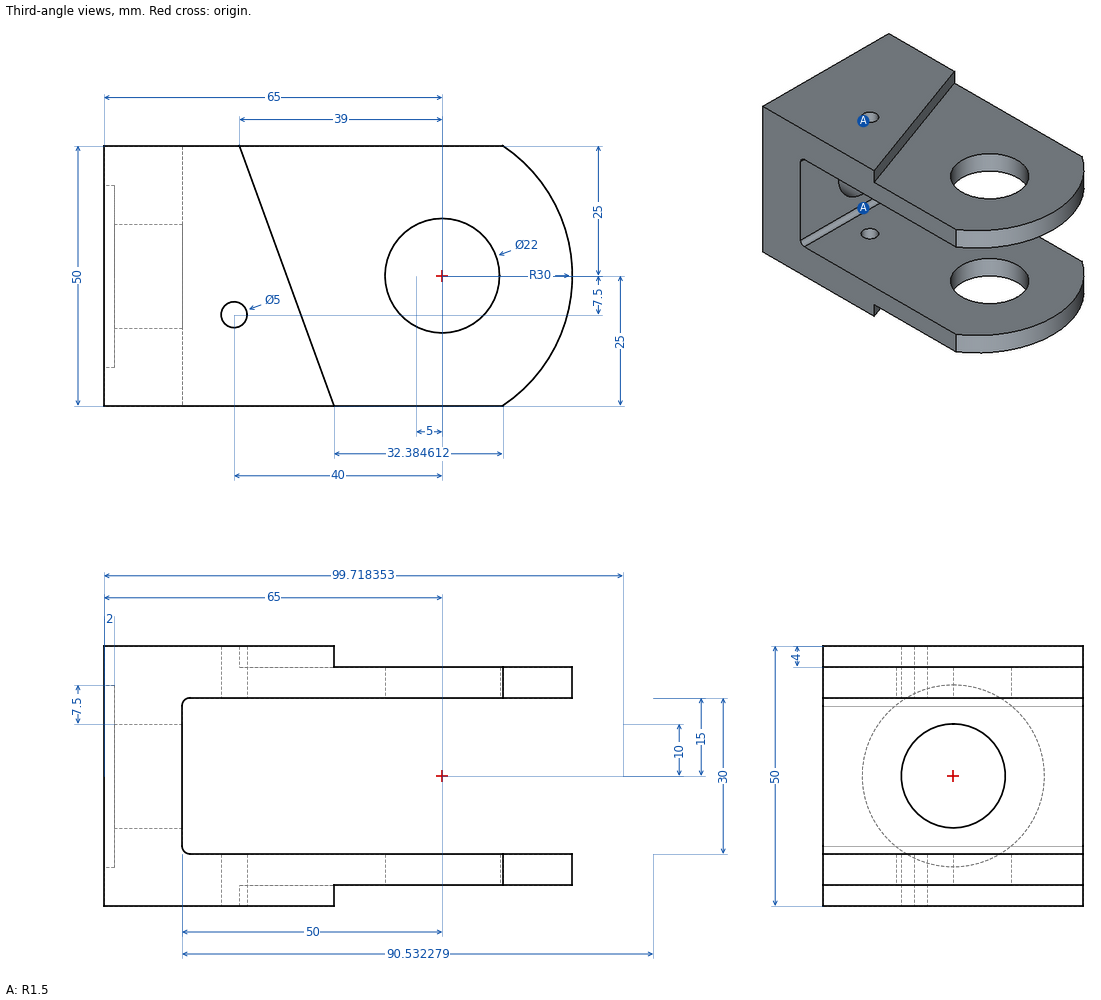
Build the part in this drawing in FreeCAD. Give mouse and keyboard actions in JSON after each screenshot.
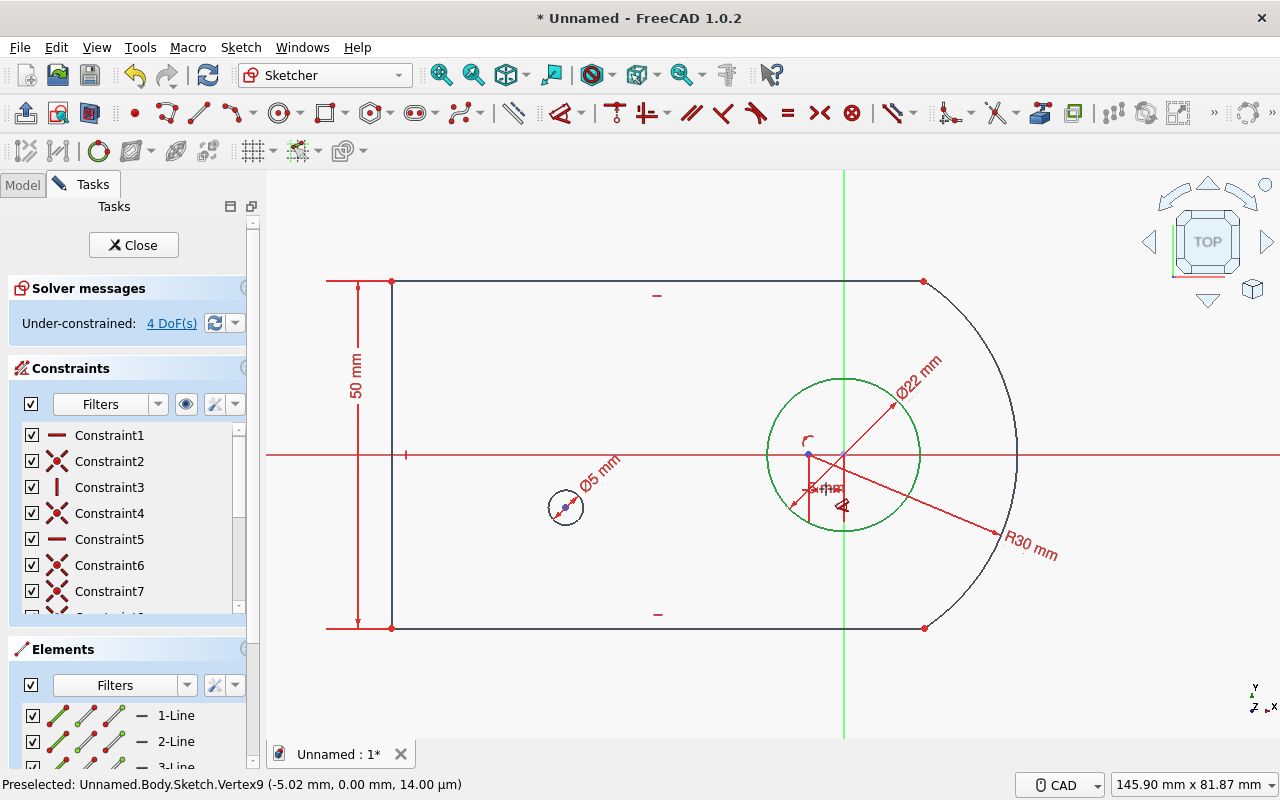
{"action": "left_click", "coordinate": [566, 508]}
{"action": "left_click", "coordinate": [705, 542]}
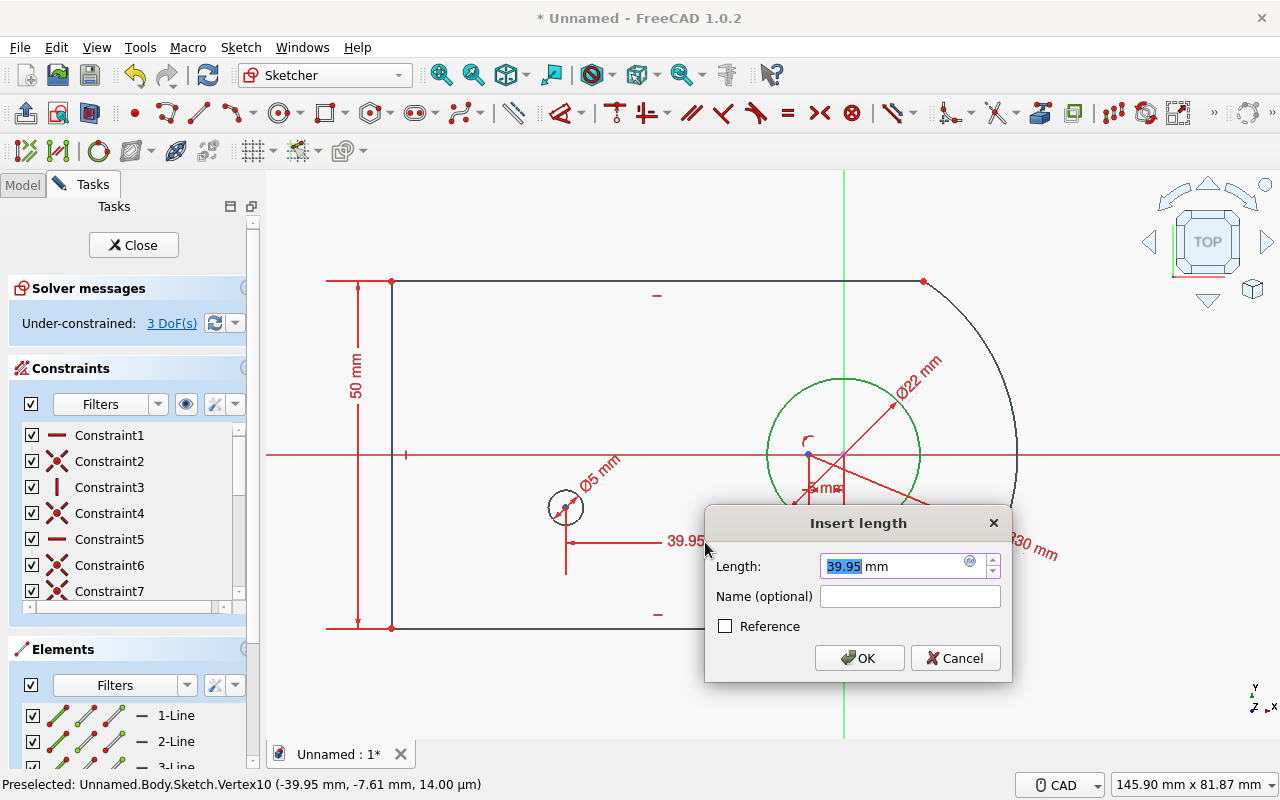
{"action": "type", "text": "40"}
{"action": "key", "text": "Return"}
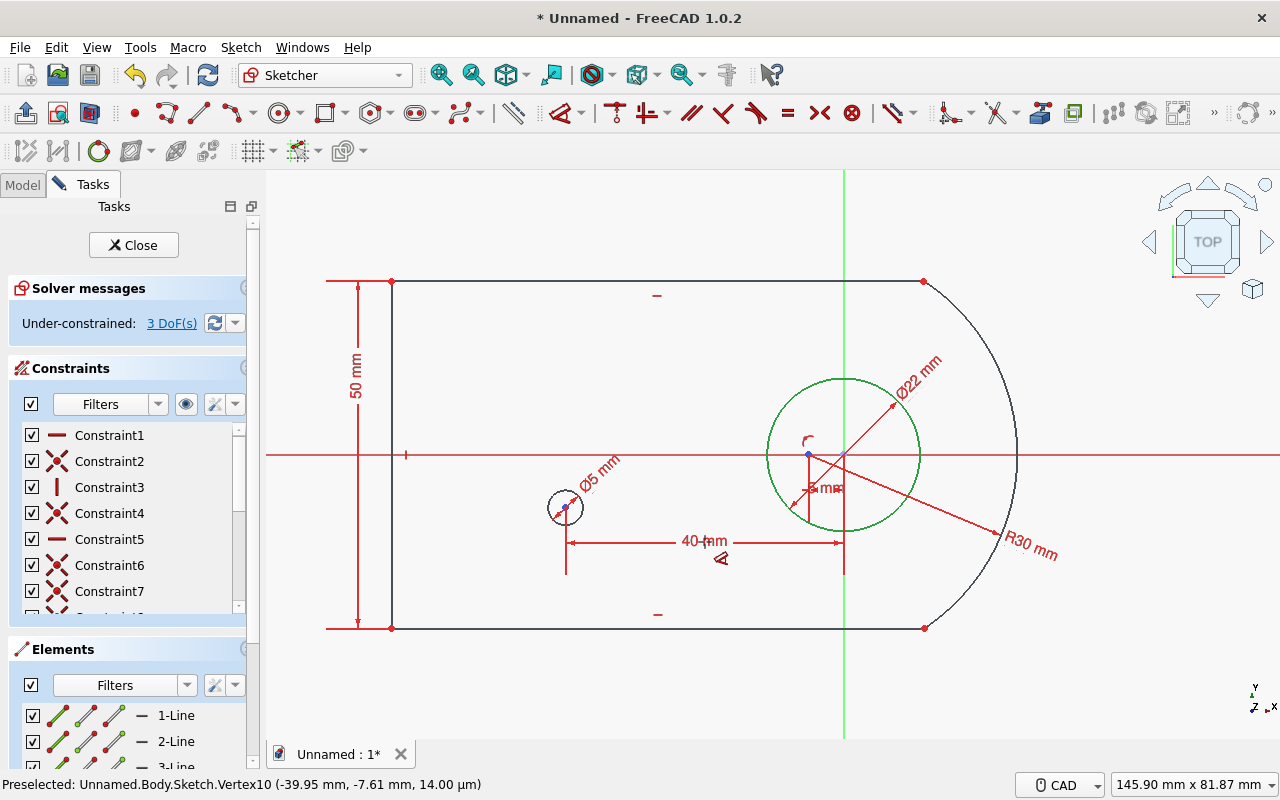
{"action": "left_click", "coordinate": [924, 281]}
{"action": "left_click", "coordinate": [958, 408]}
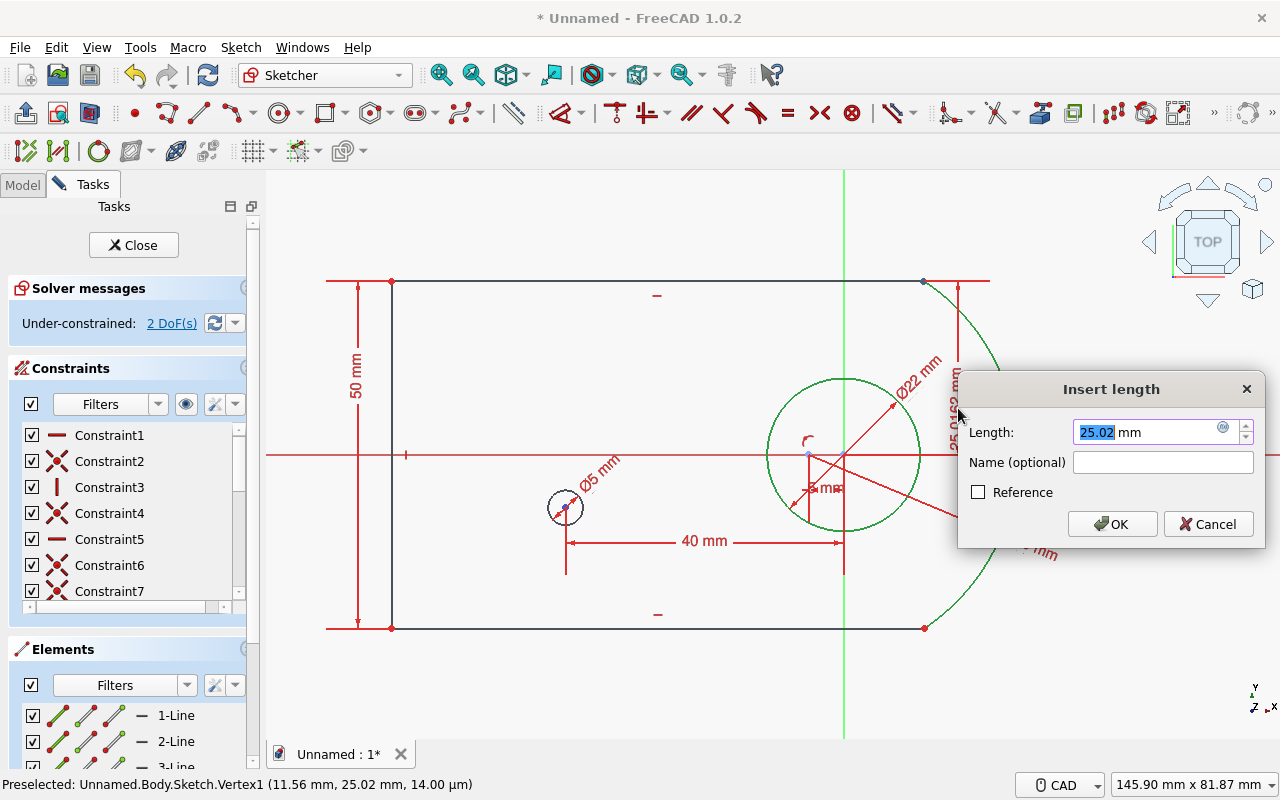
{"action": "type", "text": "25"}
{"action": "key", "text": "Return"}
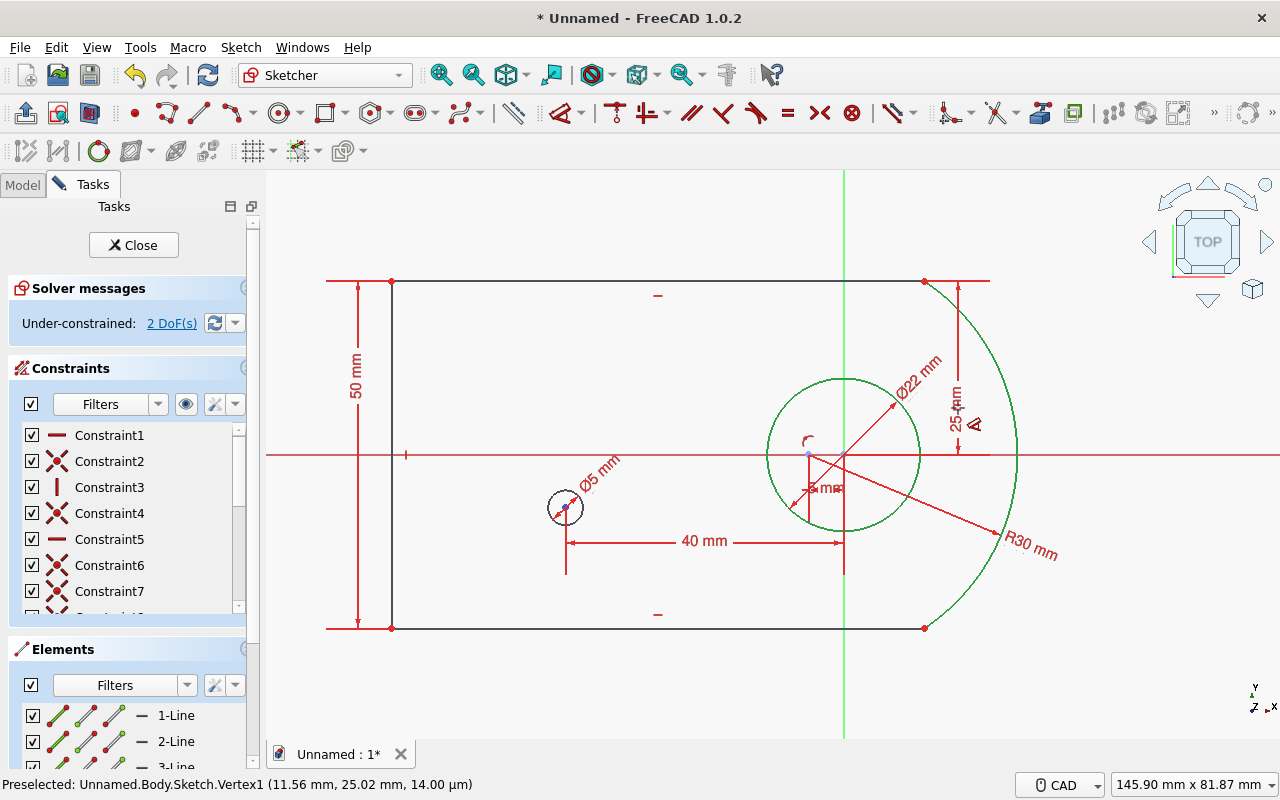
{"action": "left_click", "coordinate": [392, 281]}
{"action": "left_click", "coordinate": [618, 247]}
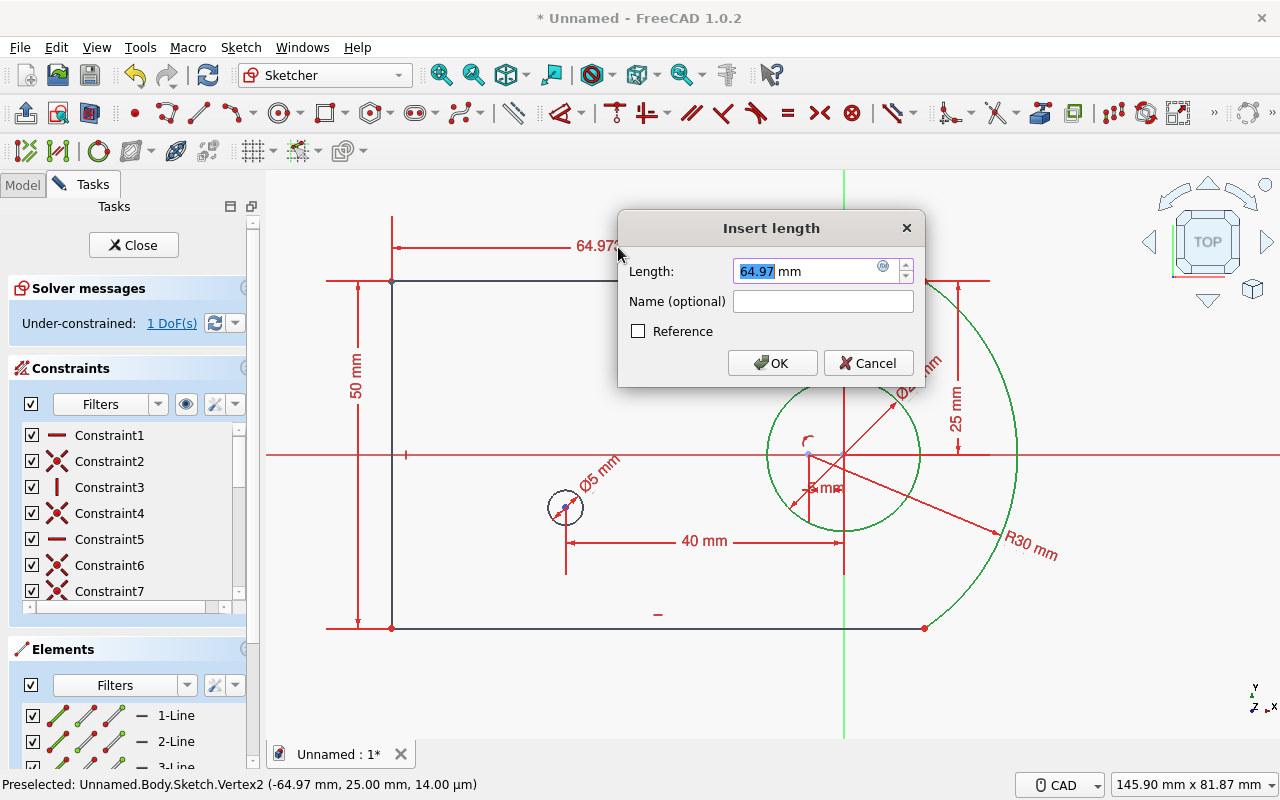
{"action": "type", "text": "65"}
{"action": "key", "text": "Return"}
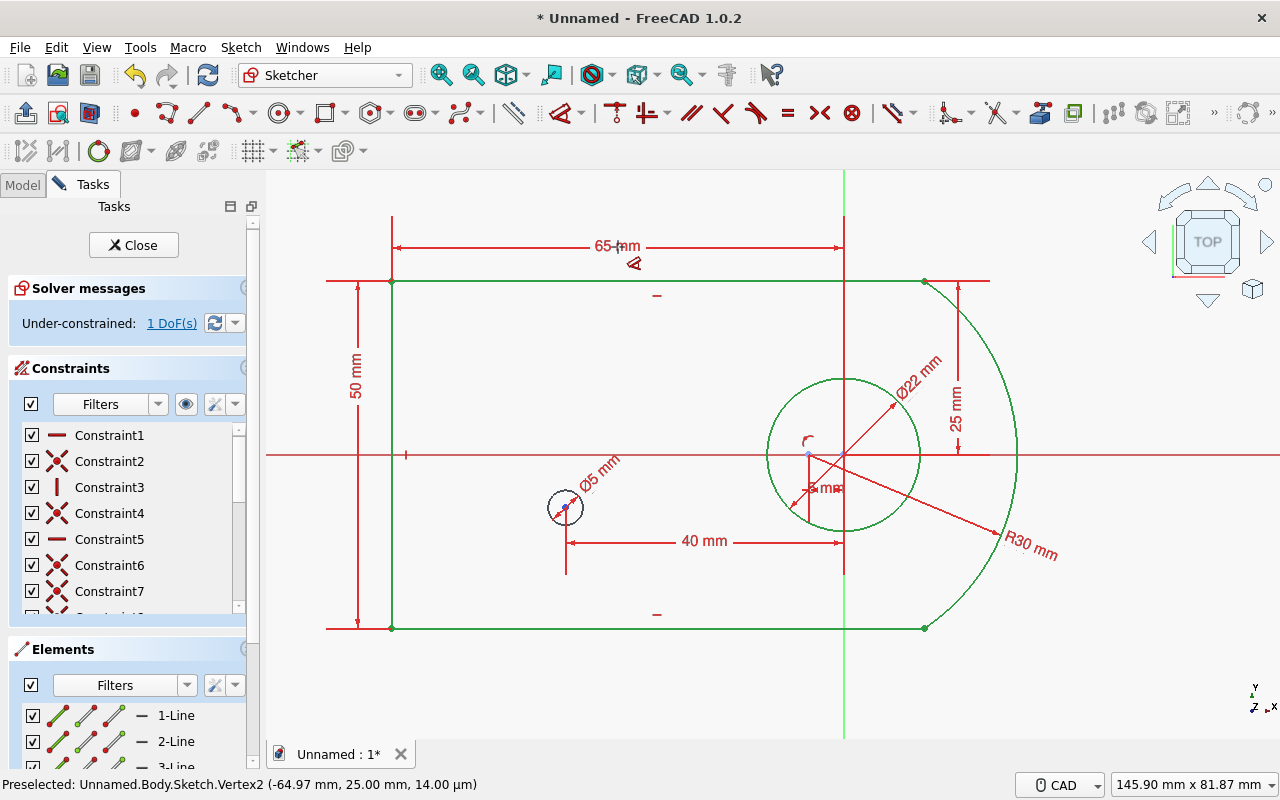
{"action": "left_click", "coordinate": [566, 508]}
{"action": "left_click", "coordinate": [532, 500]}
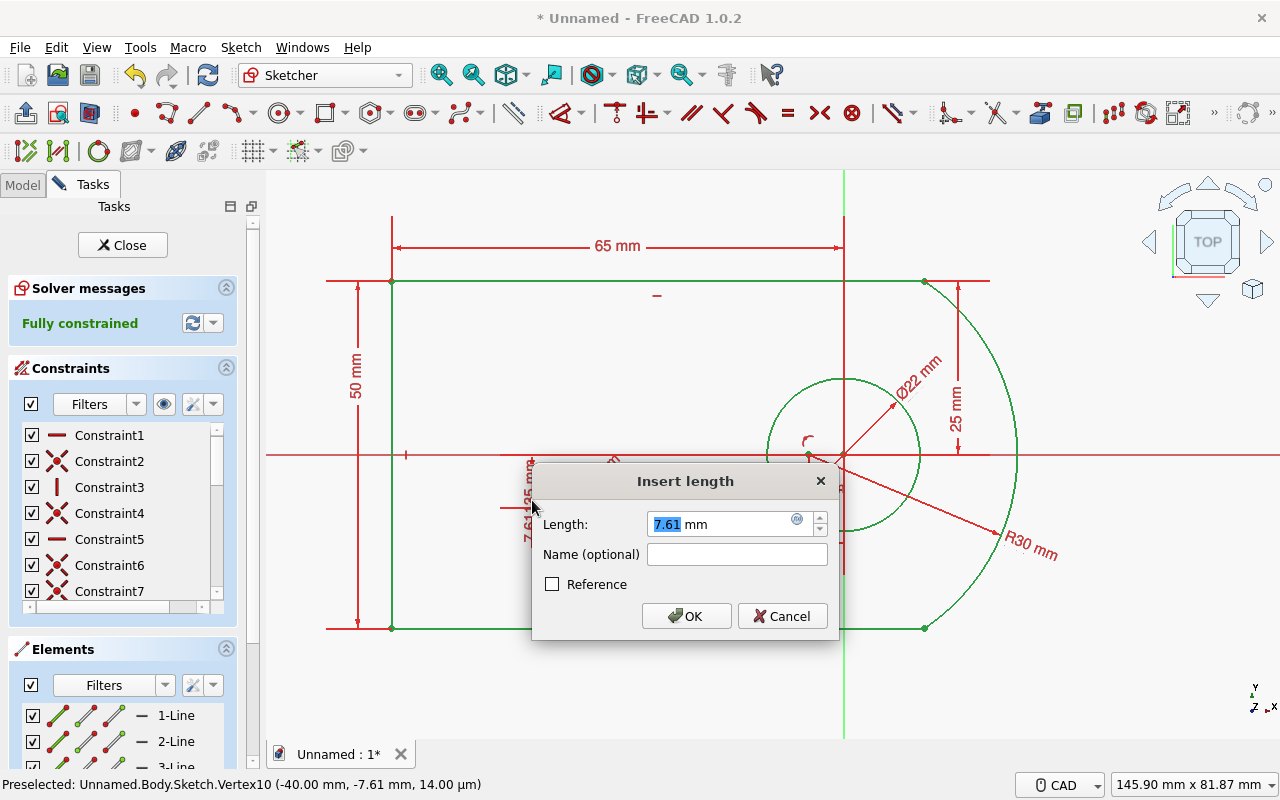
{"action": "type", "text": "7.5"}
{"action": "key", "text": "Return"}
{"action": "key", "text": "Escape"}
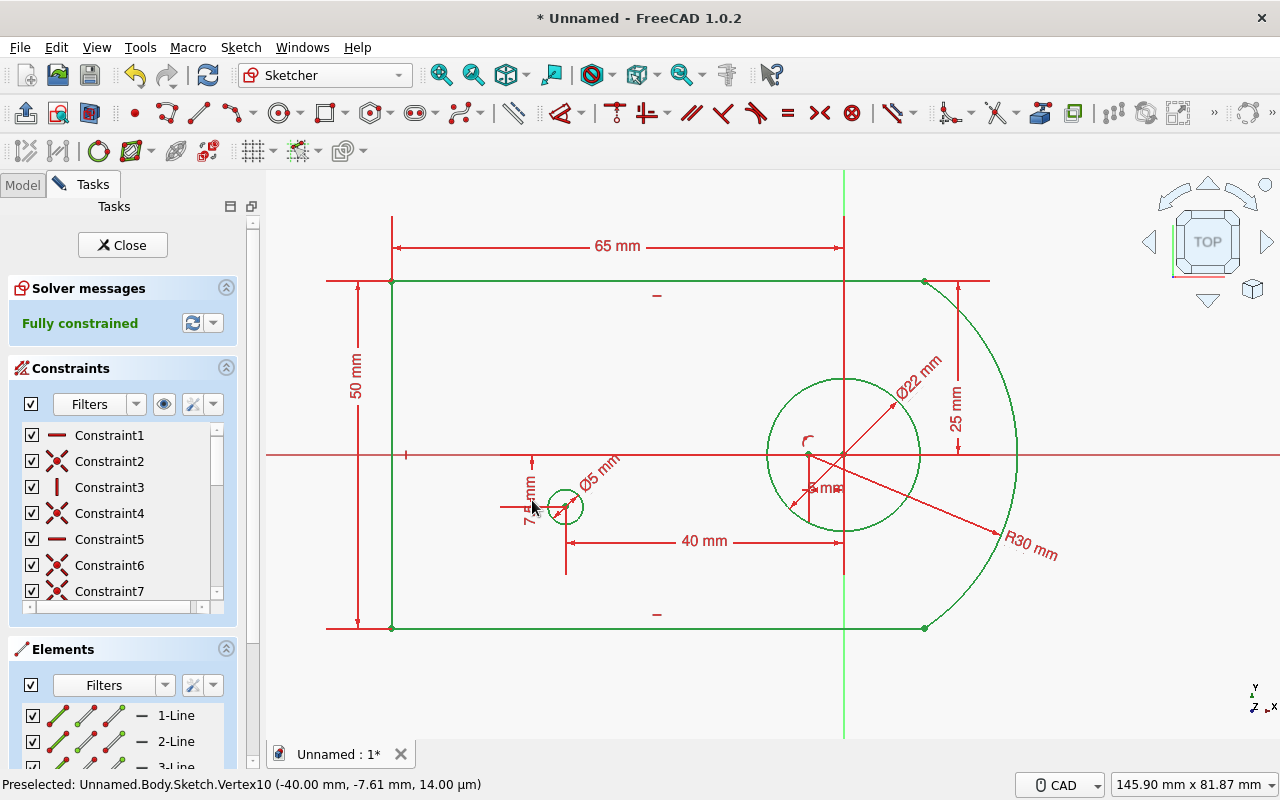
{"action": "left_click", "coordinate": [123, 245]}